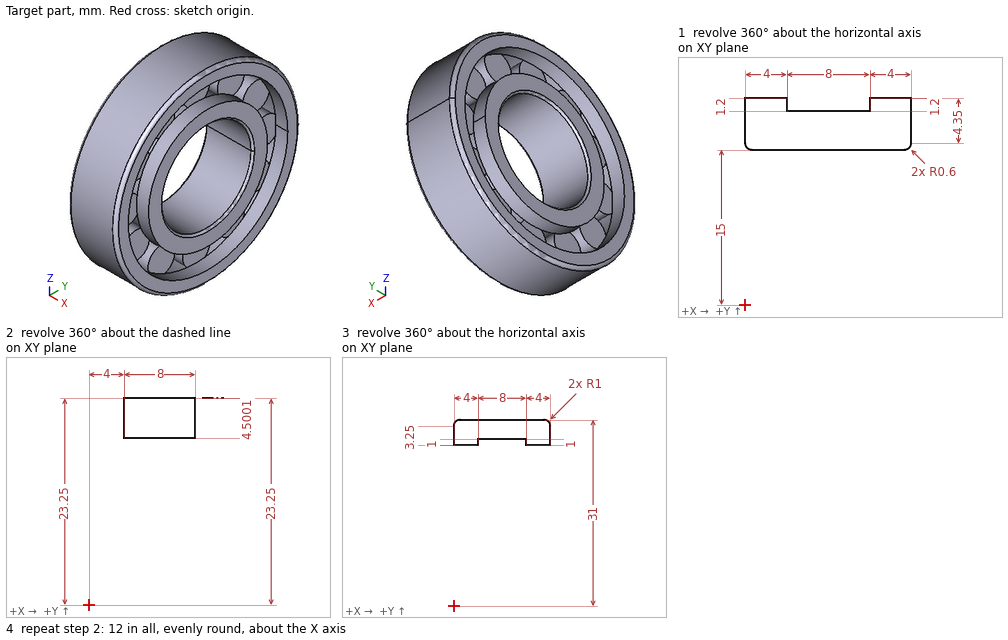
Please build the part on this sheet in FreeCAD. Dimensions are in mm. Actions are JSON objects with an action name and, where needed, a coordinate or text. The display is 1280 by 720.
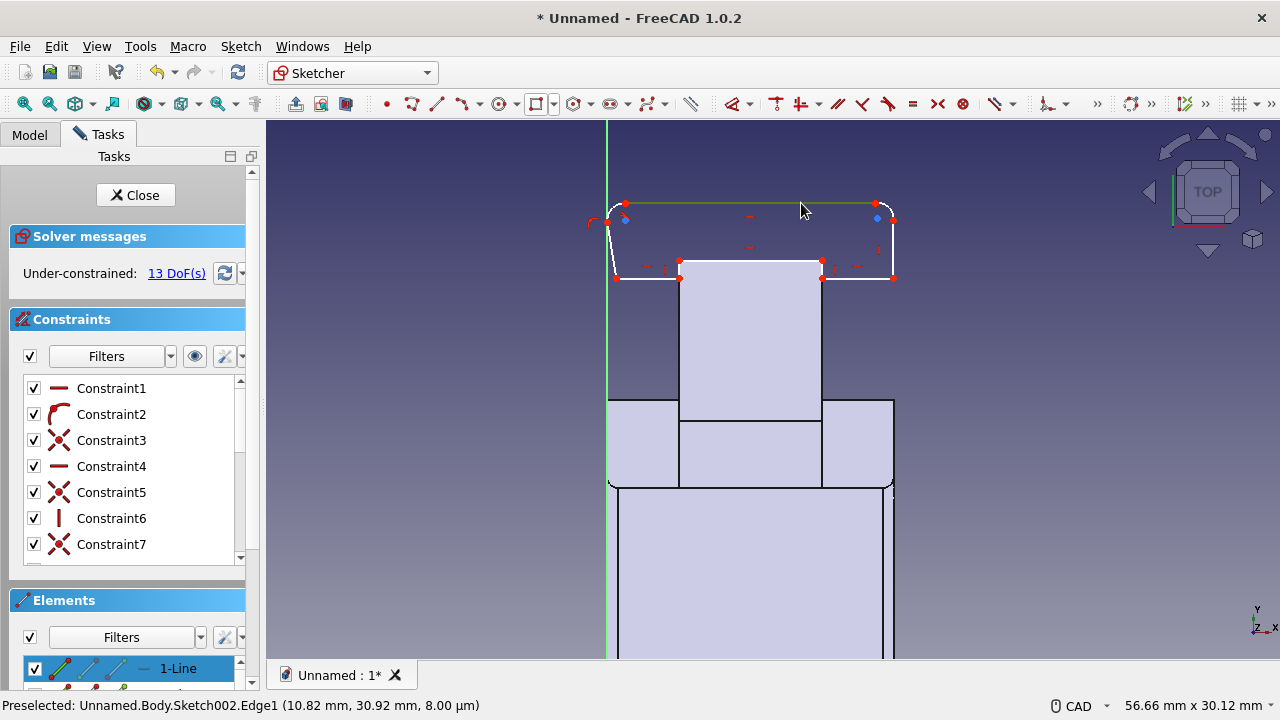
{"action": "left_click", "coordinate": [889, 208]}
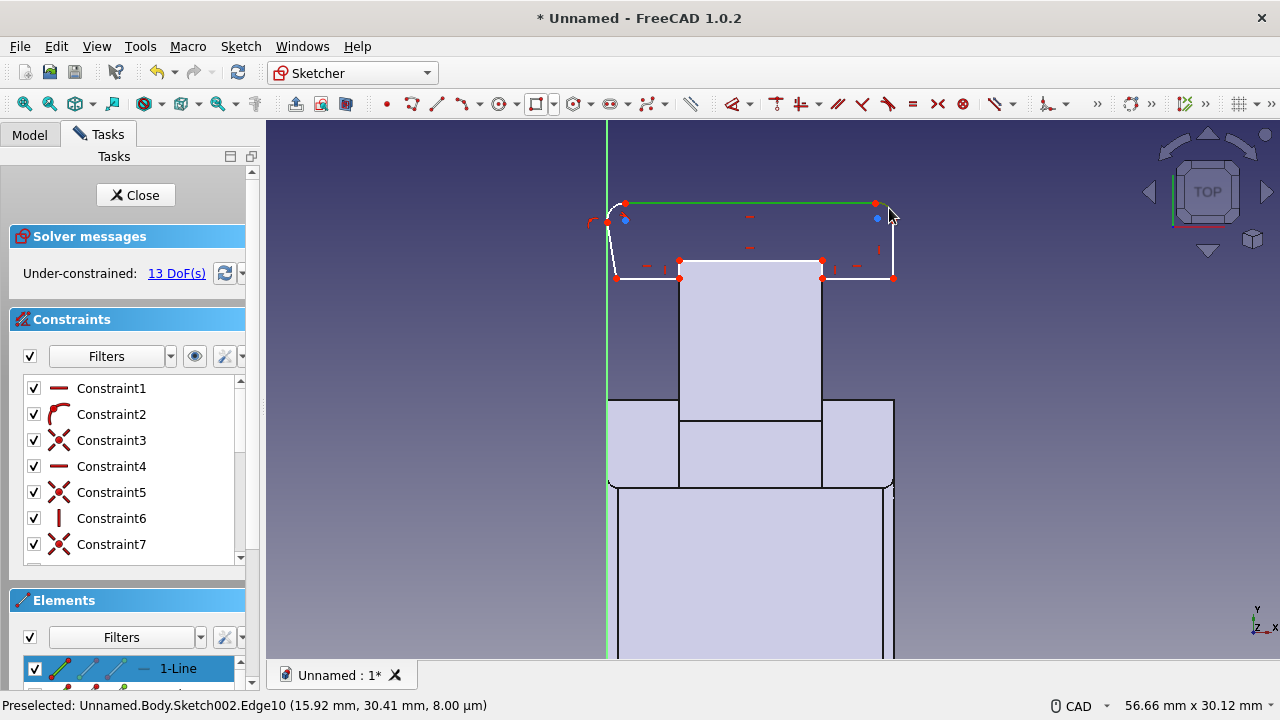
{"action": "left_click", "coordinate": [888, 104]}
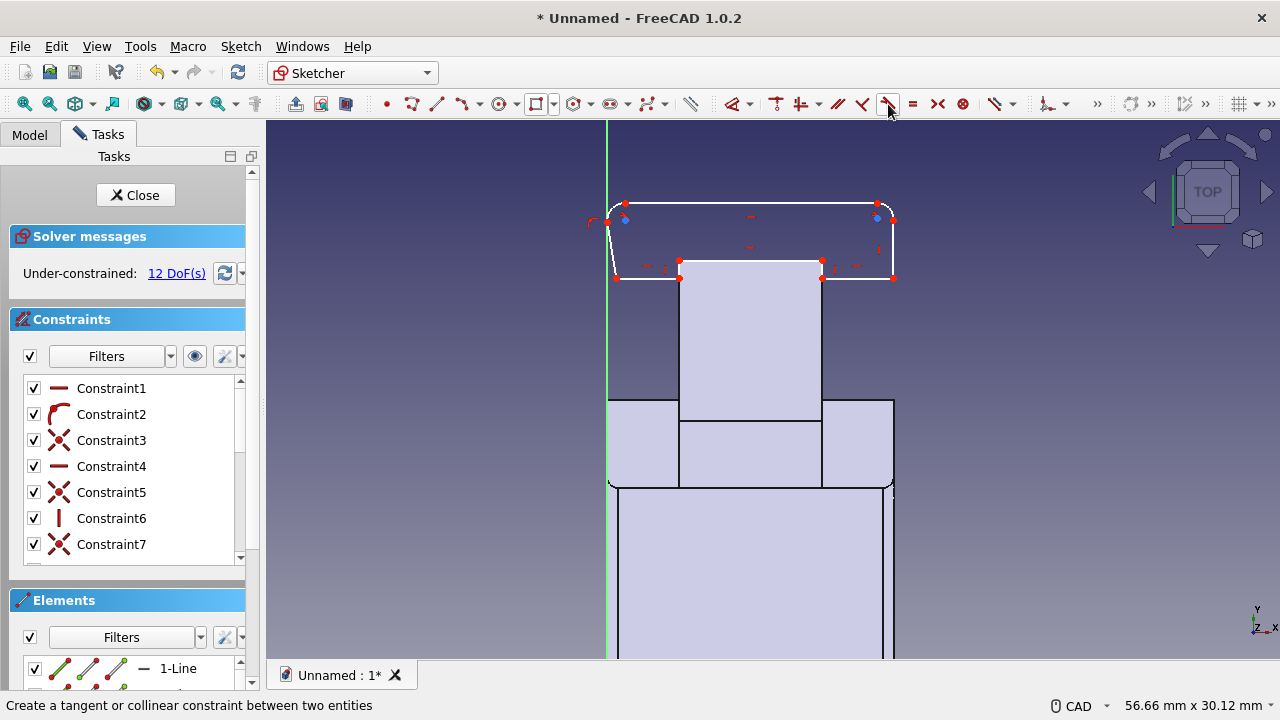
{"action": "left_click", "coordinate": [610, 240]}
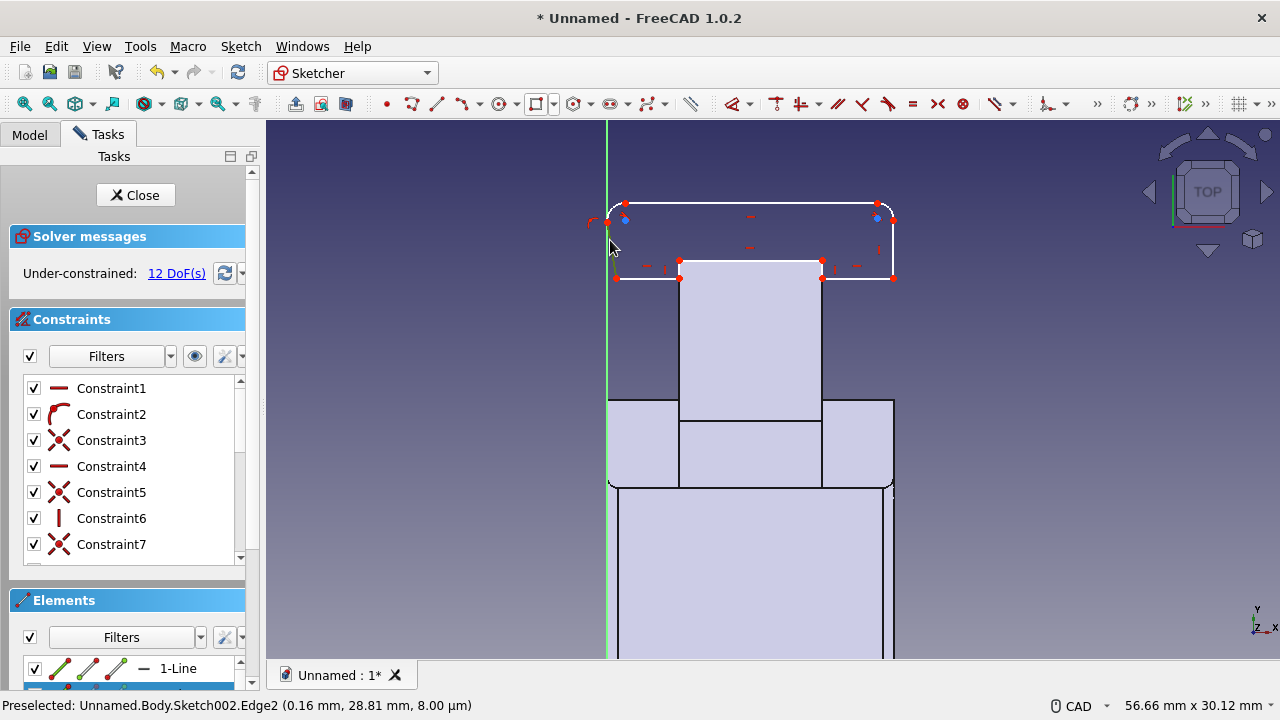
{"action": "scroll", "coordinate": [609, 214], "scroll_direction": "up", "scroll_amount": 3}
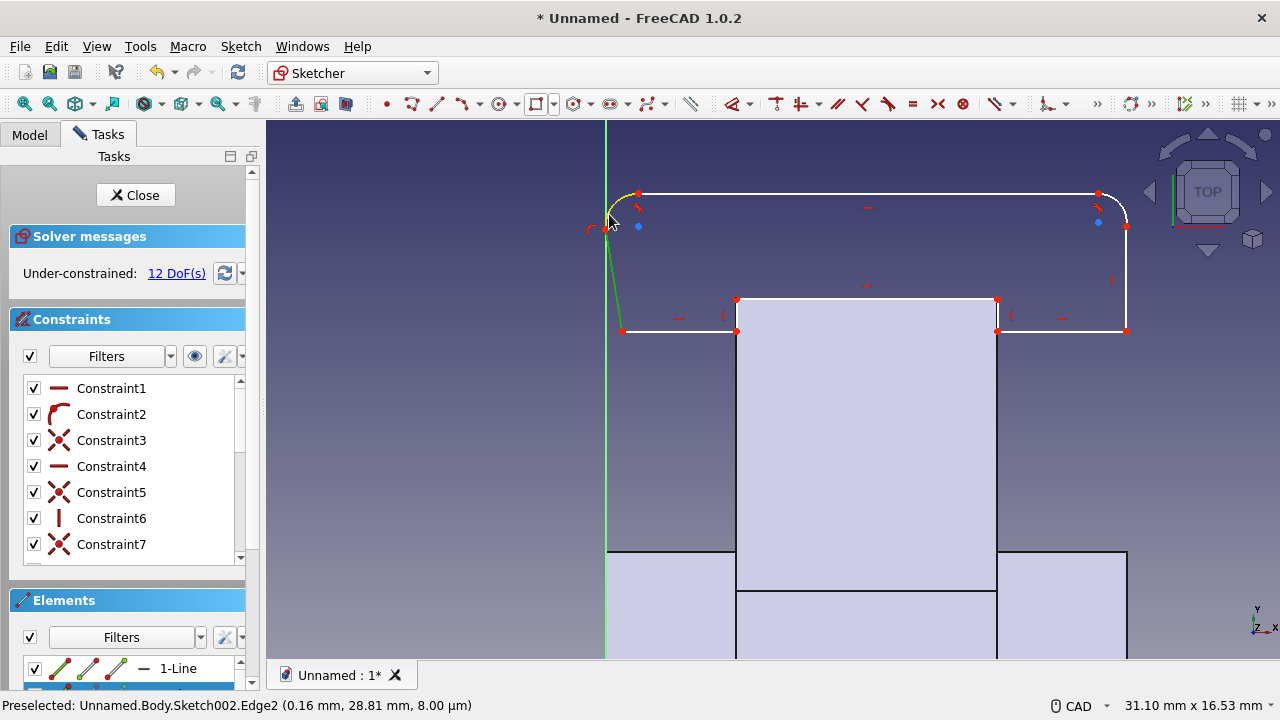
{"action": "left_click", "coordinate": [608, 214]}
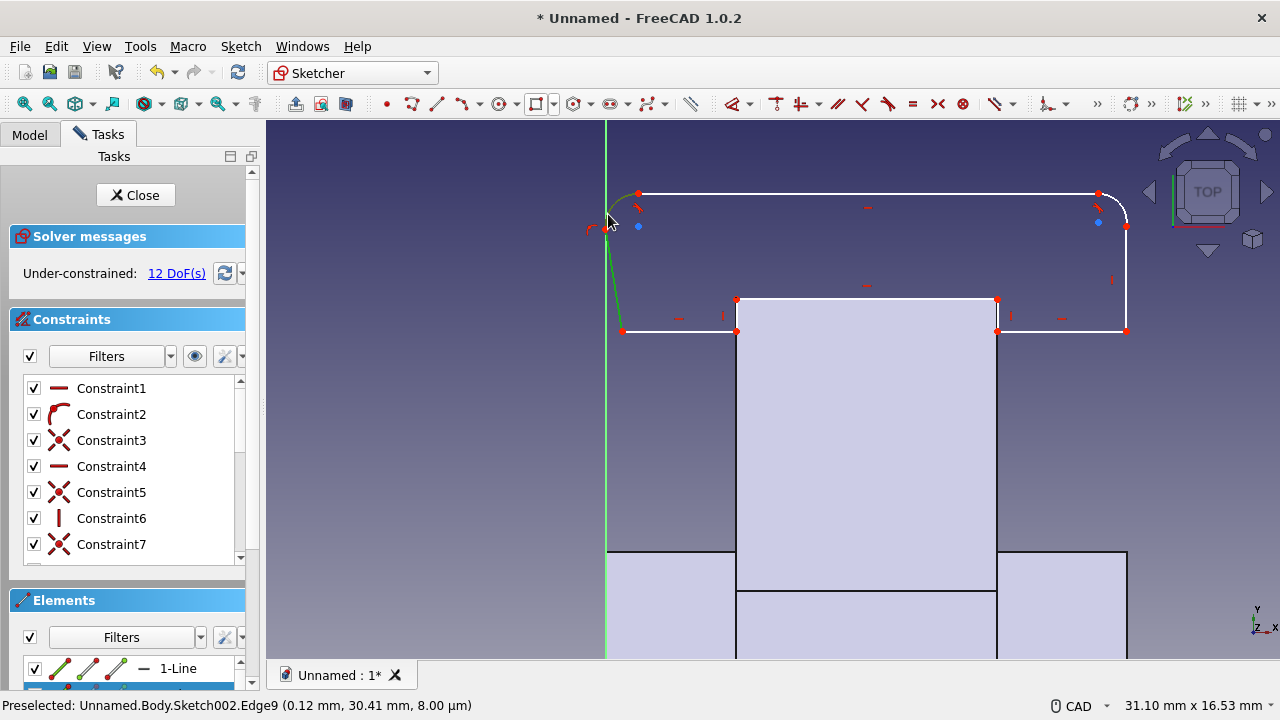
{"action": "left_click", "coordinate": [888, 104]}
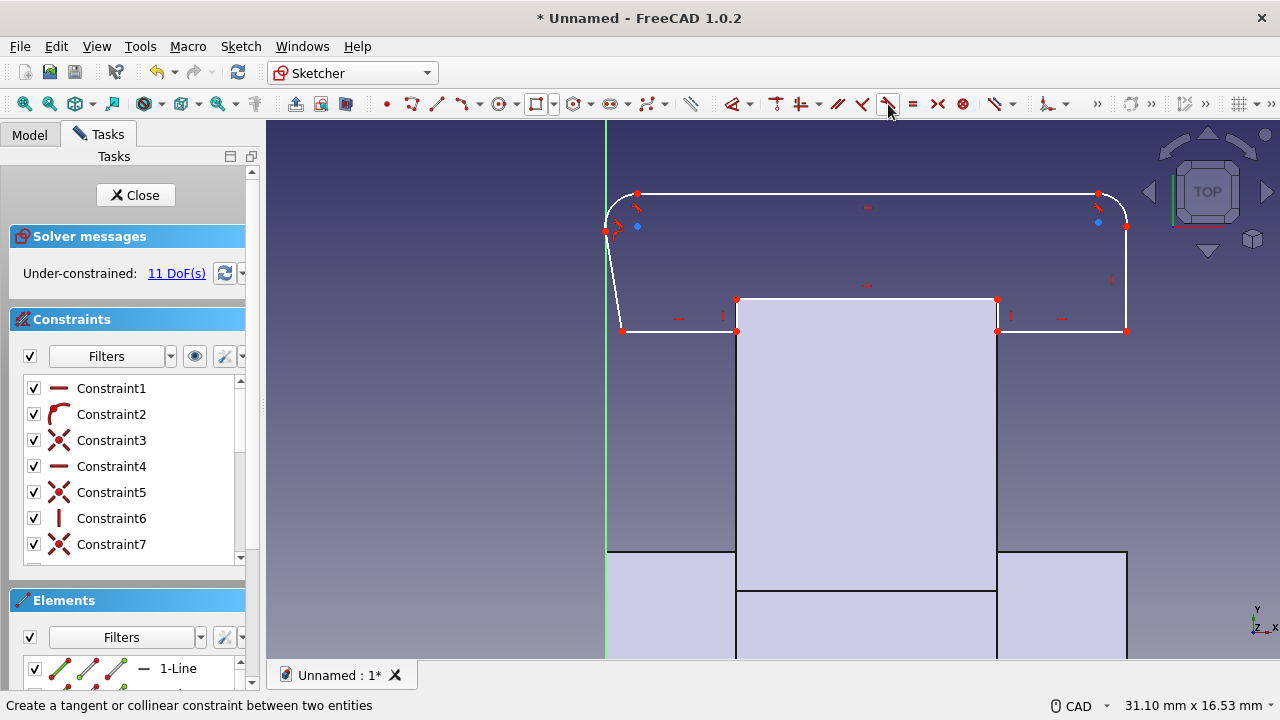
{"action": "scroll", "coordinate": [610, 211], "scroll_direction": "down", "scroll_amount": 5}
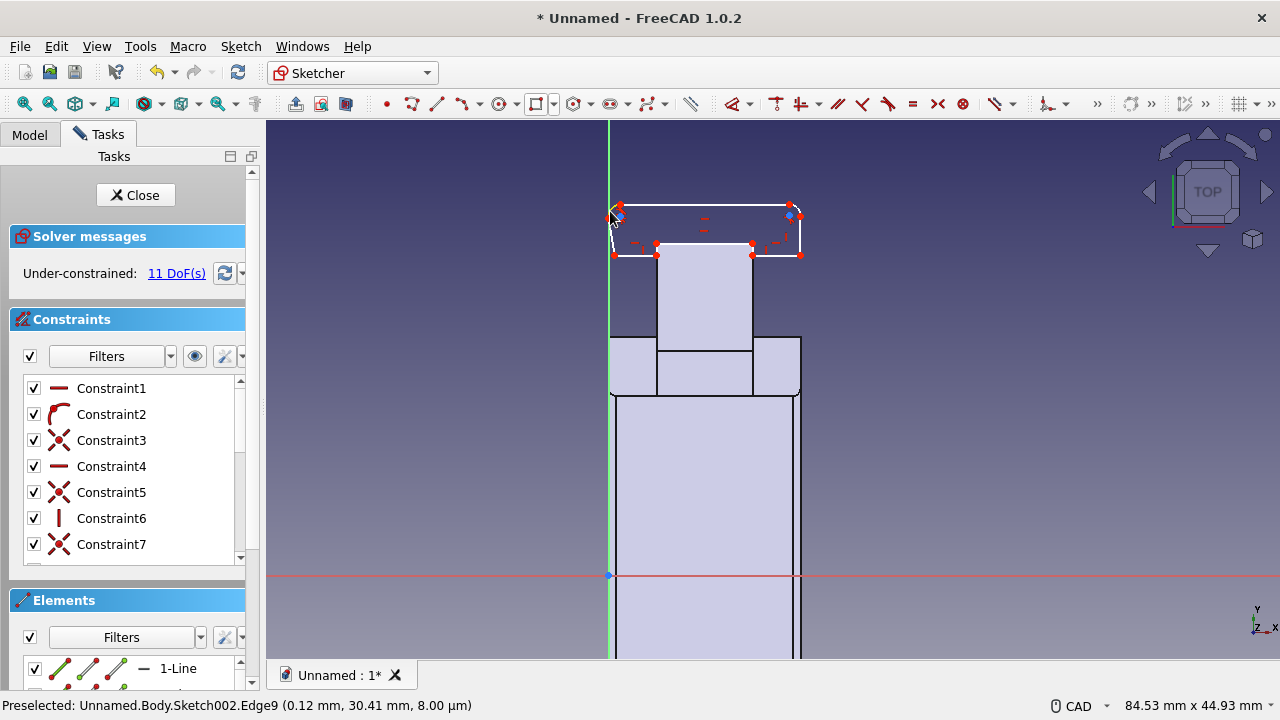
{"action": "left_click", "coordinate": [800, 244]}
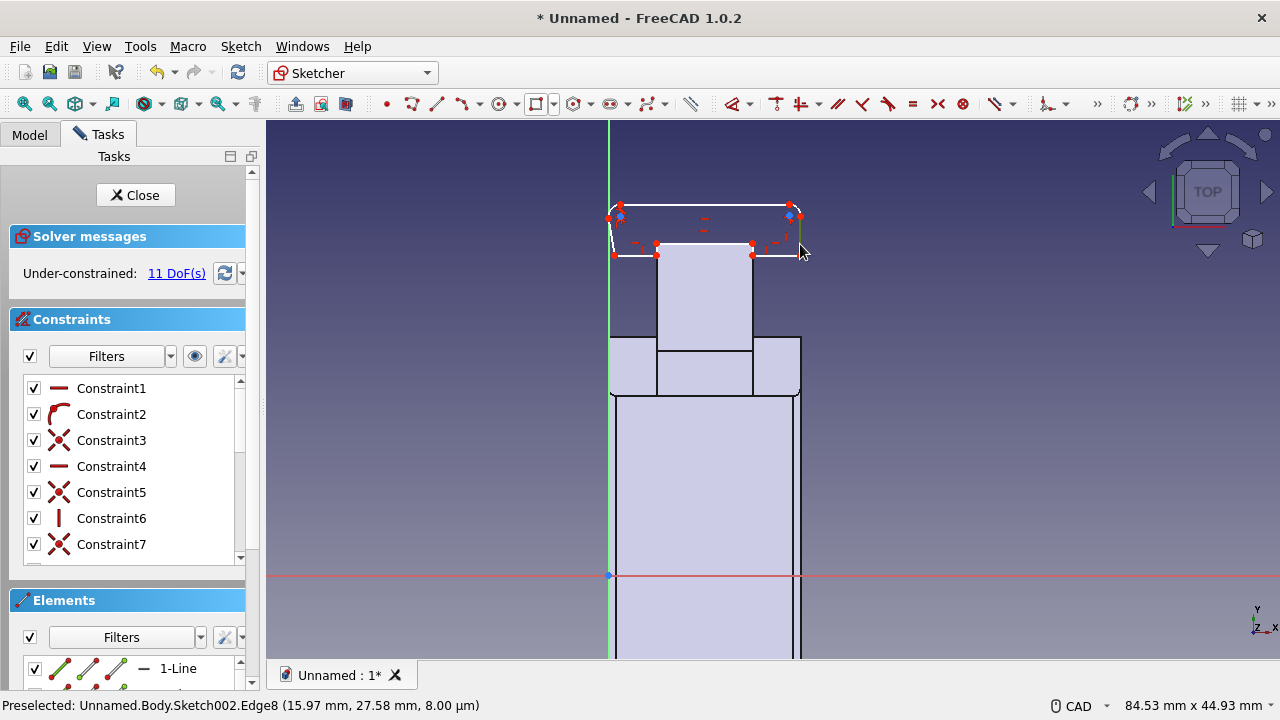
{"action": "scroll", "coordinate": [798, 208], "scroll_direction": "up", "scroll_amount": 3}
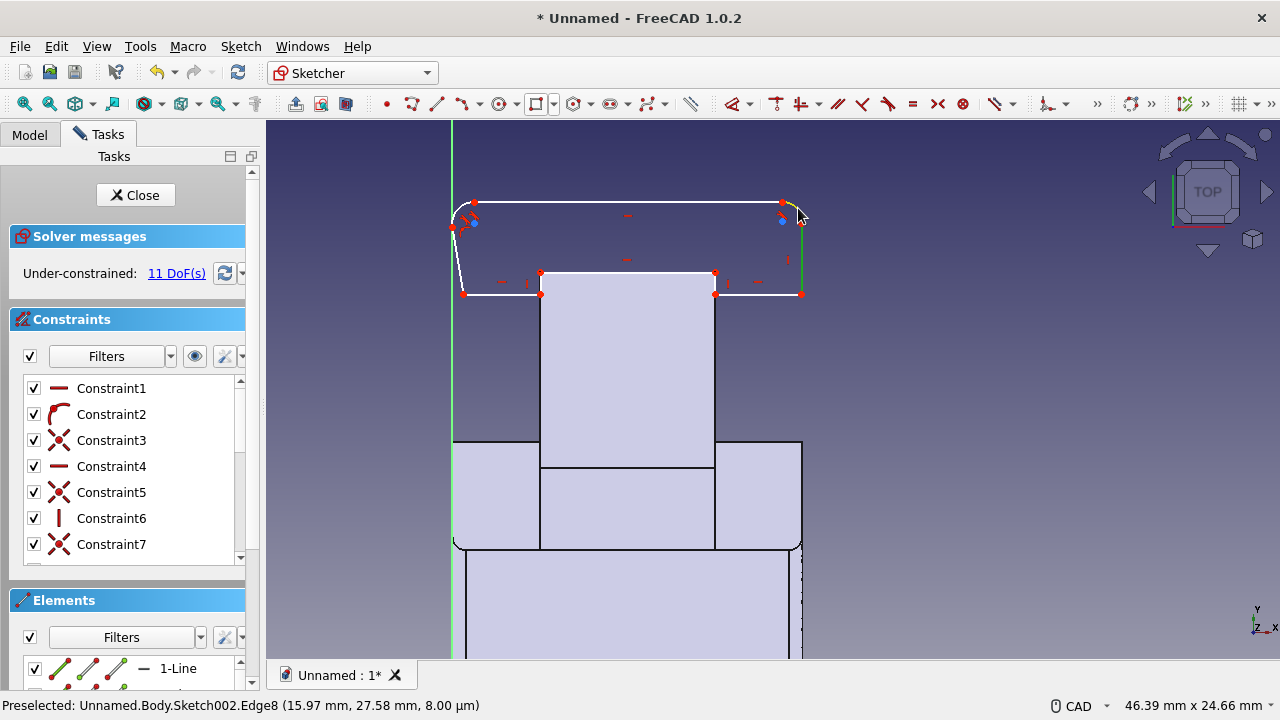
{"action": "left_click", "coordinate": [797, 209]}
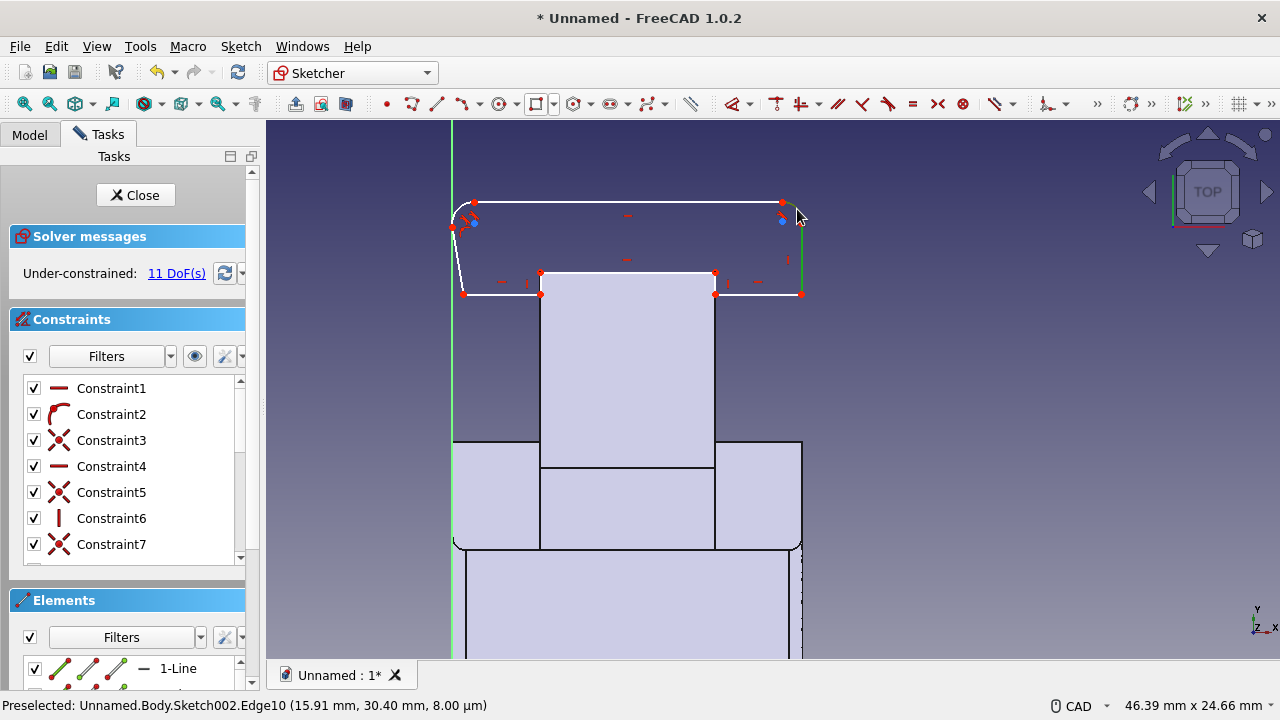
{"action": "left_click", "coordinate": [888, 104]}